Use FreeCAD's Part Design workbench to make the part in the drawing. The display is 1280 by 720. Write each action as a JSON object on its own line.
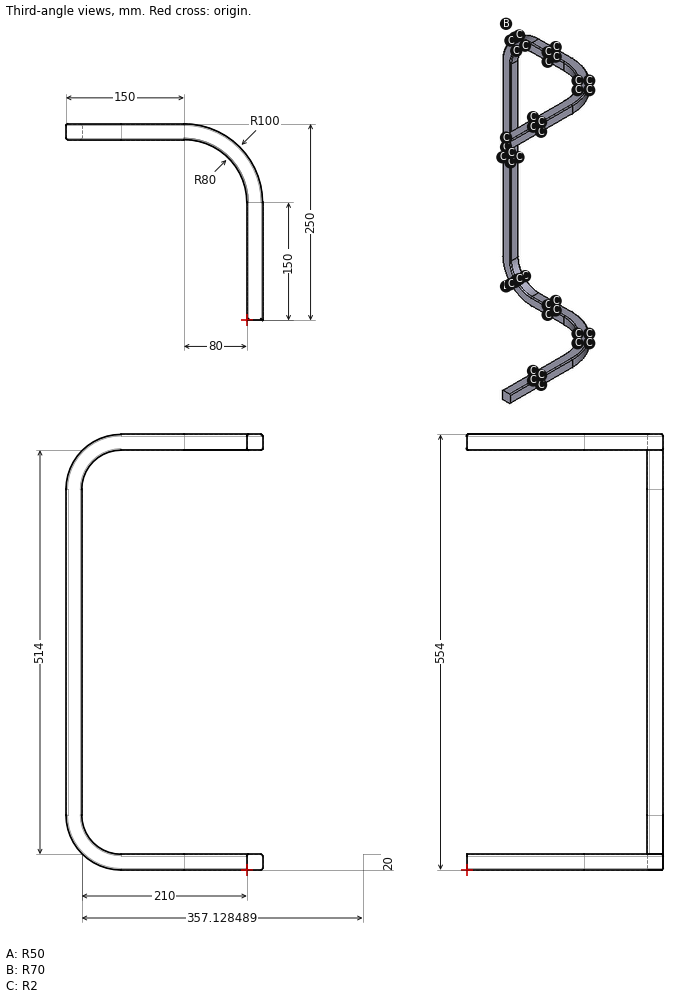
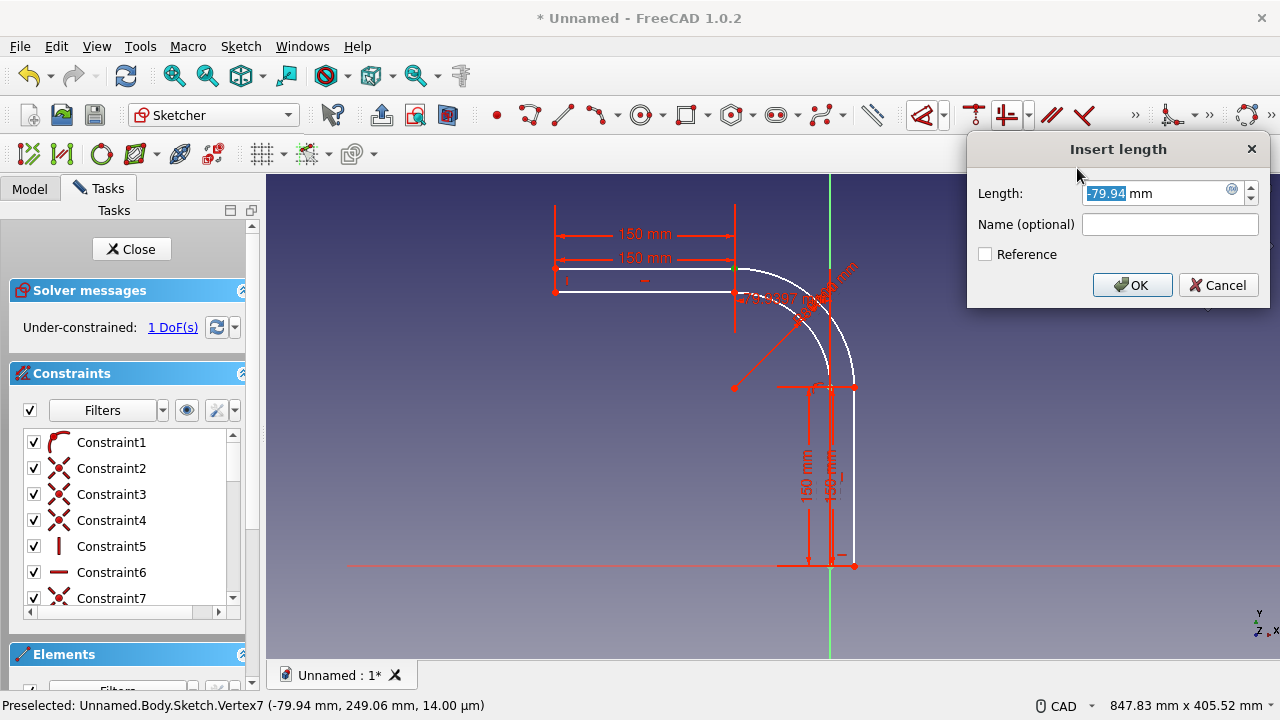
{"action": "type", "text": "-80"}
{"action": "key", "text": "Return"}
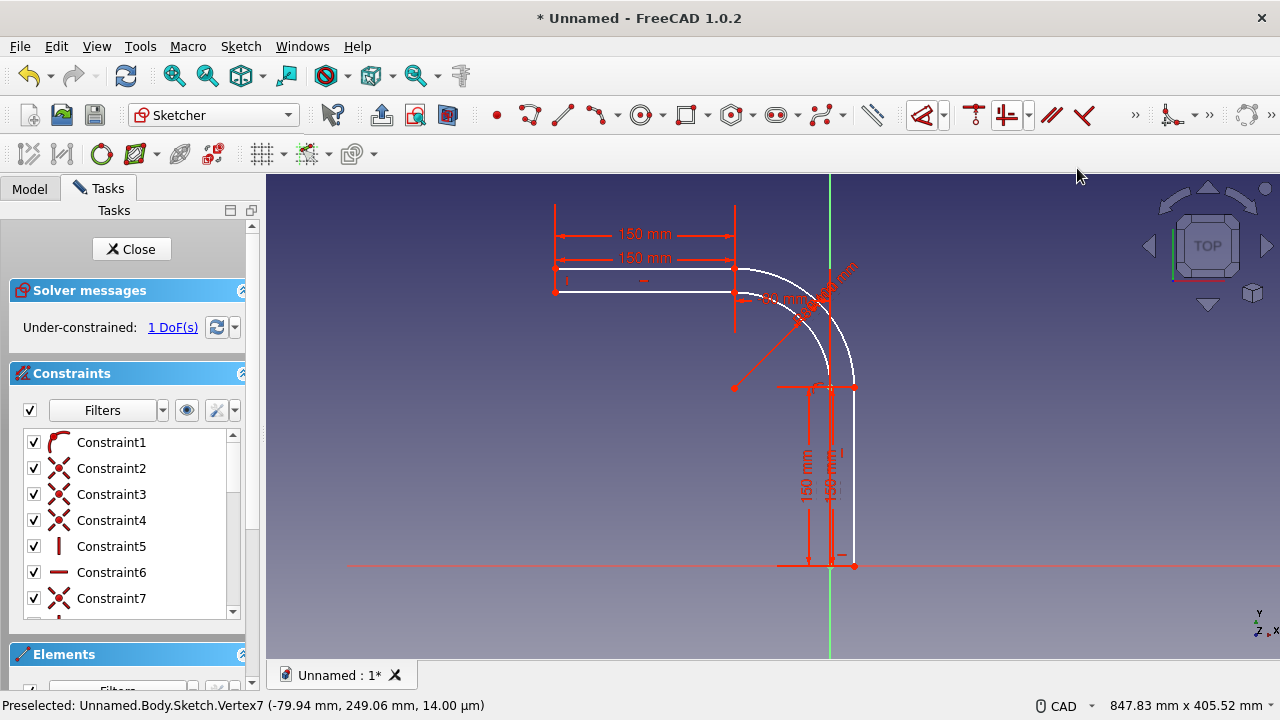
{"action": "left_click", "coordinate": [735, 269]}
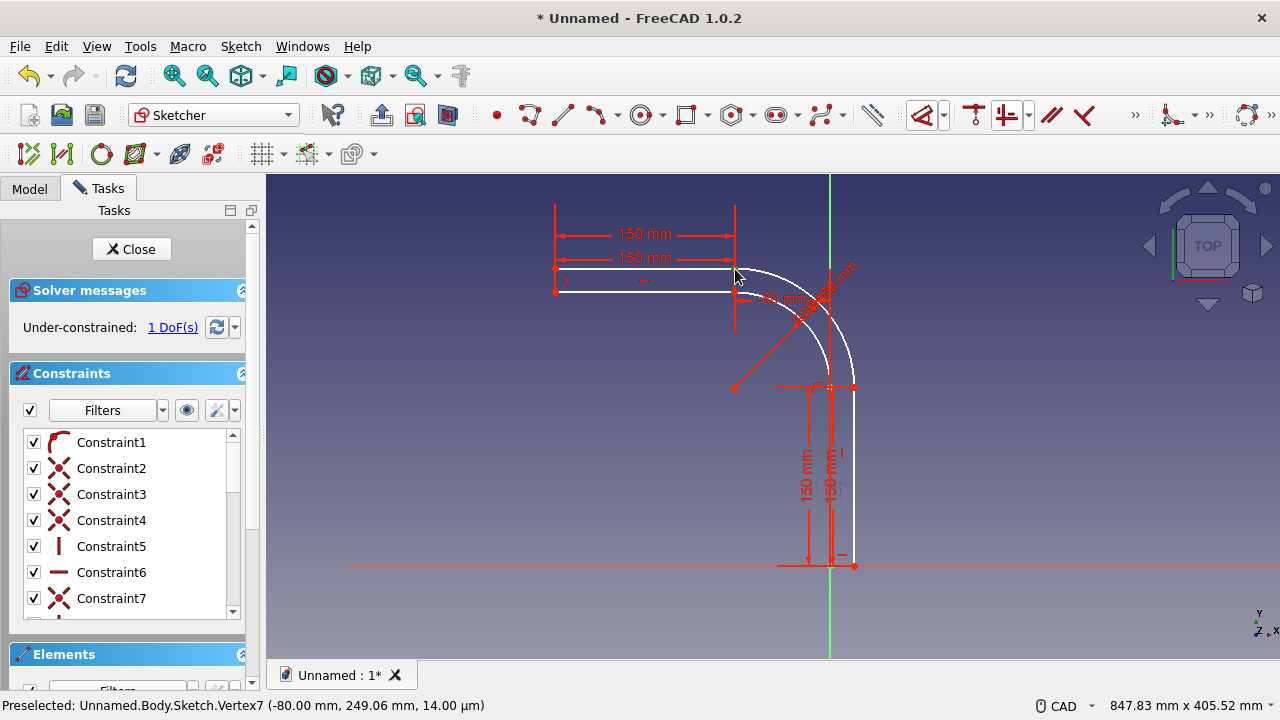
{"action": "key", "text": "i"}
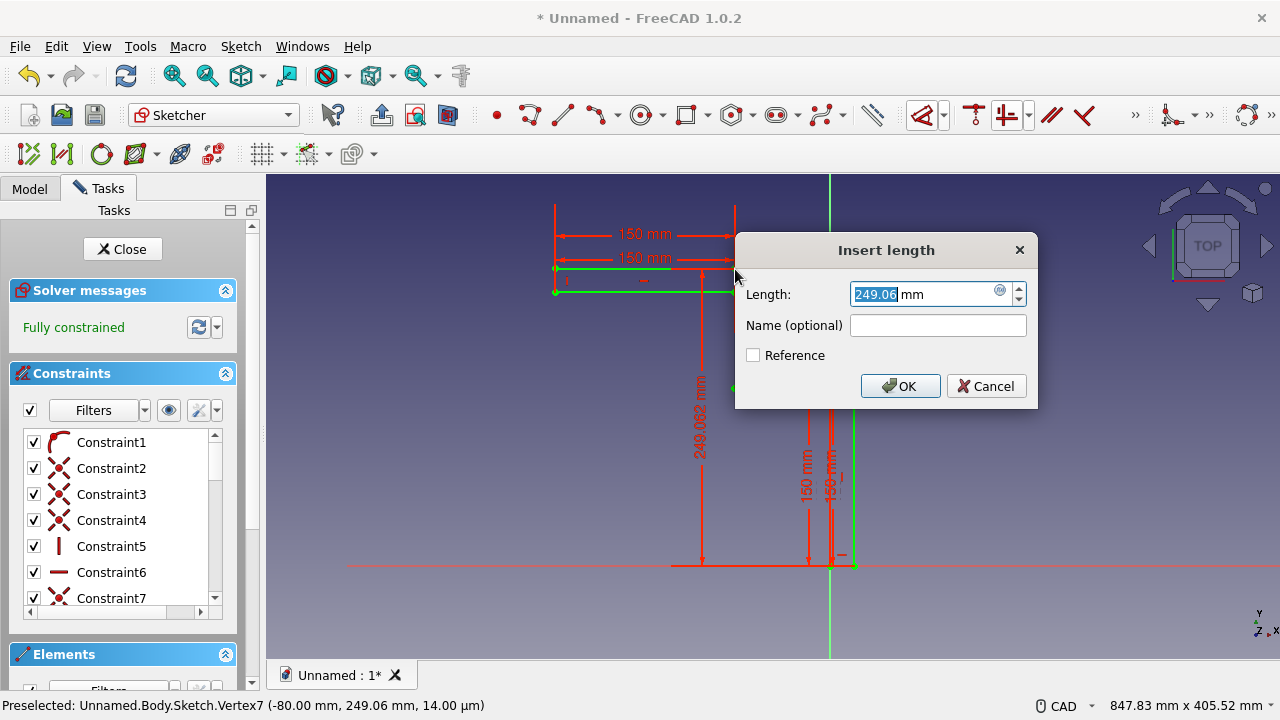
{"action": "type", "text": "250"}
{"action": "key", "text": "Return"}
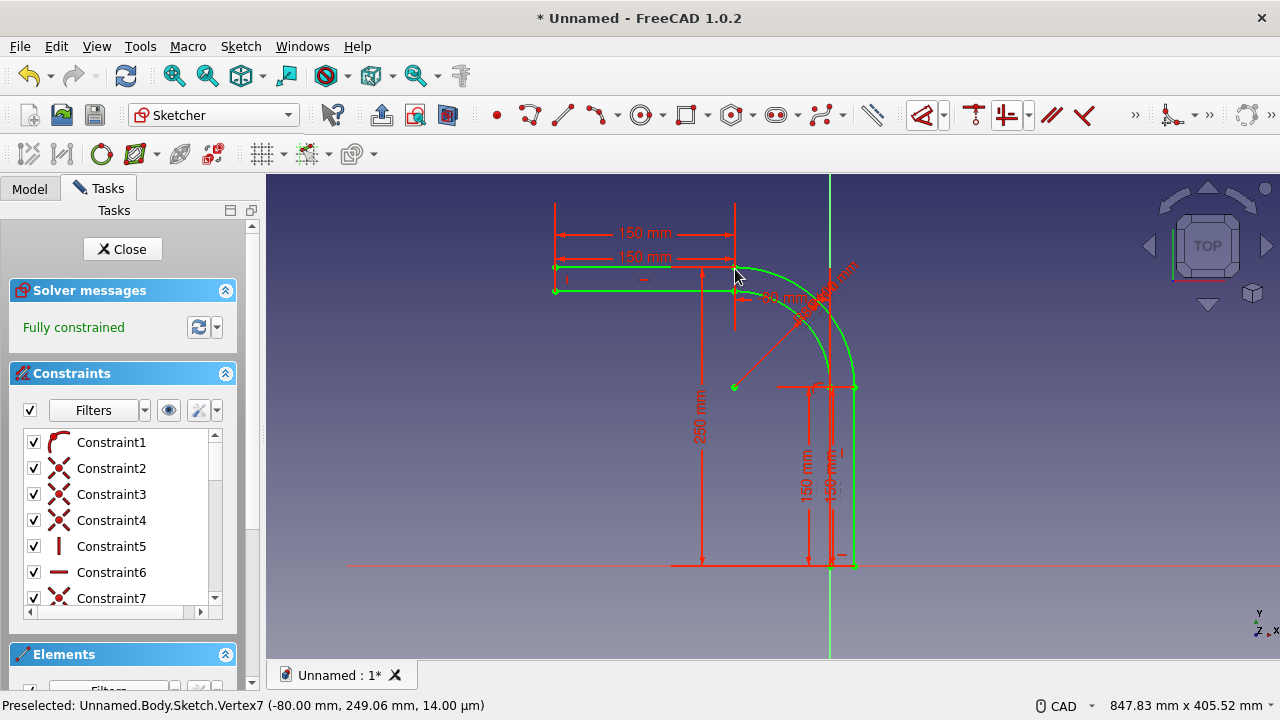
{"action": "left_click", "coordinate": [123, 249]}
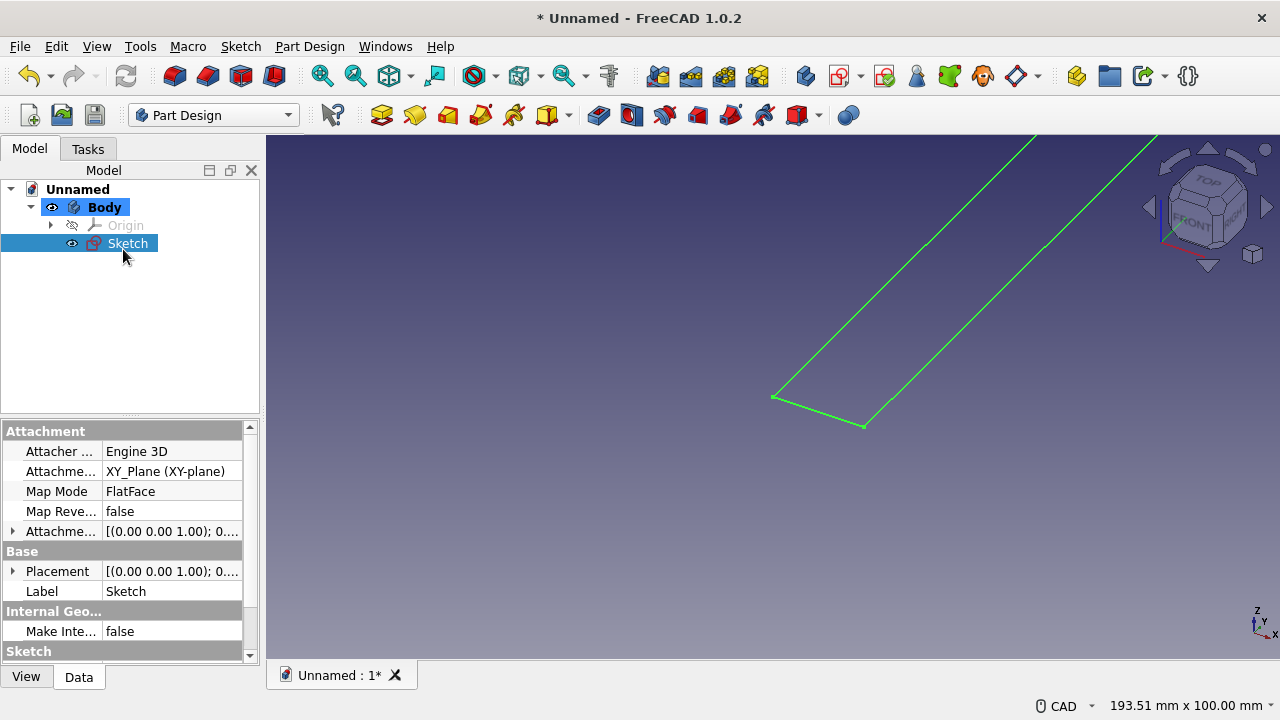
{"action": "left_click", "coordinate": [382, 116]}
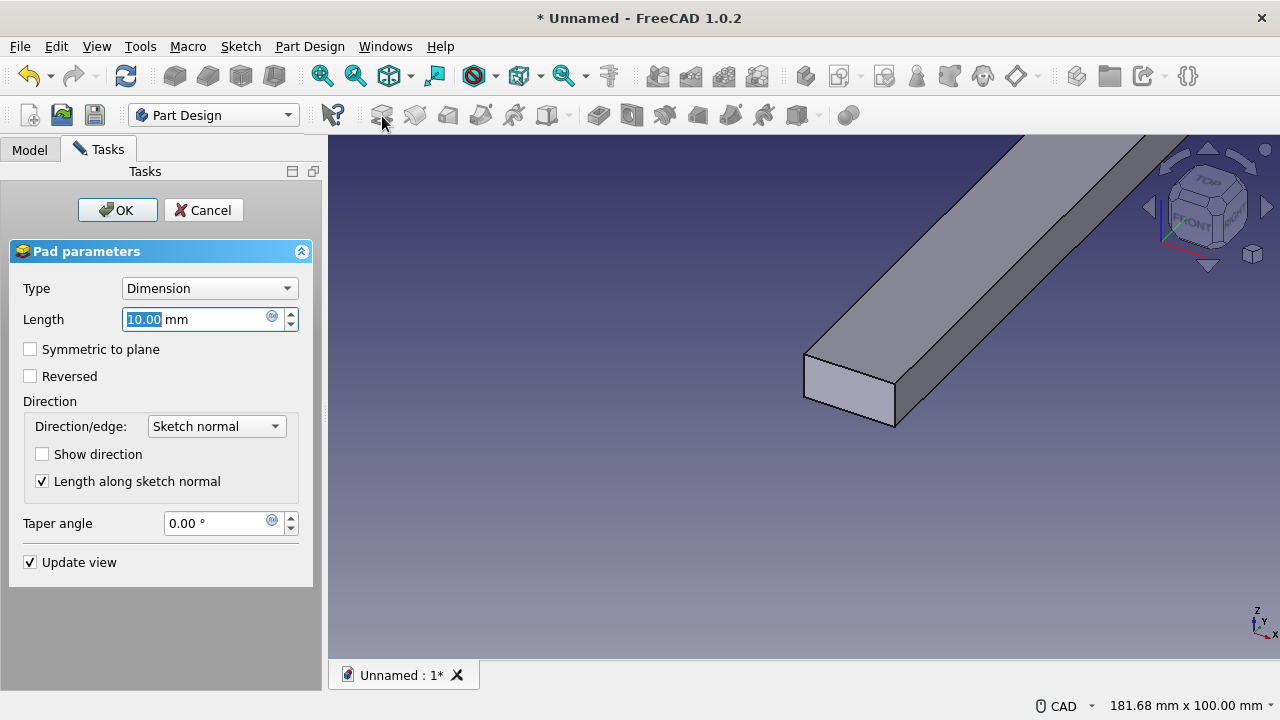
{"action": "type", "text": "554"}
{"action": "key", "text": "Tab"}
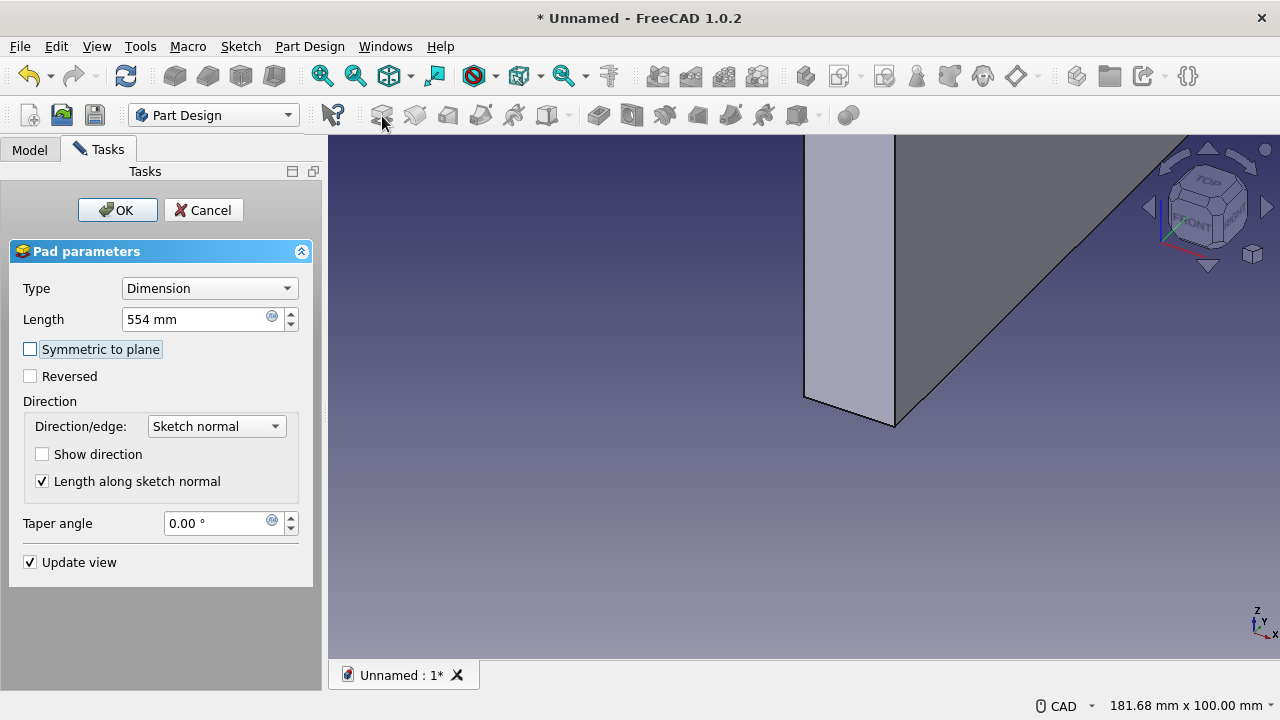
{"action": "left_click", "coordinate": [118, 210]}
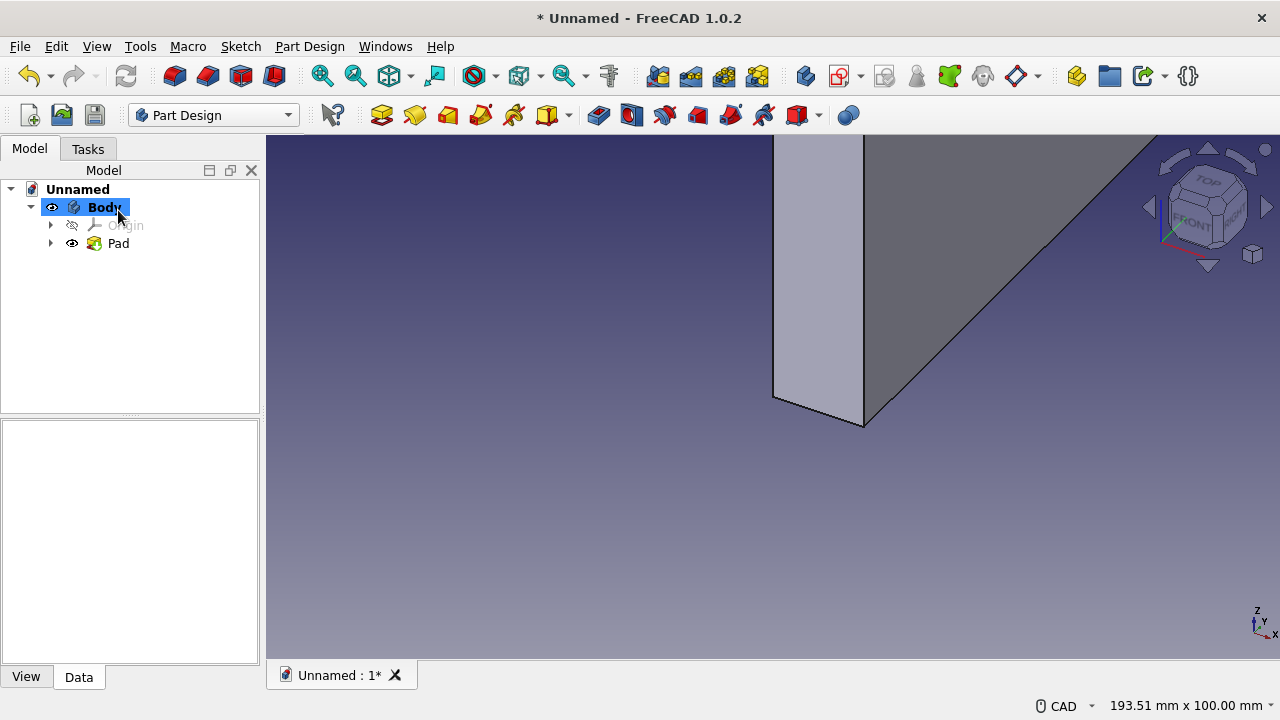
{"action": "left_click", "coordinate": [323, 76]}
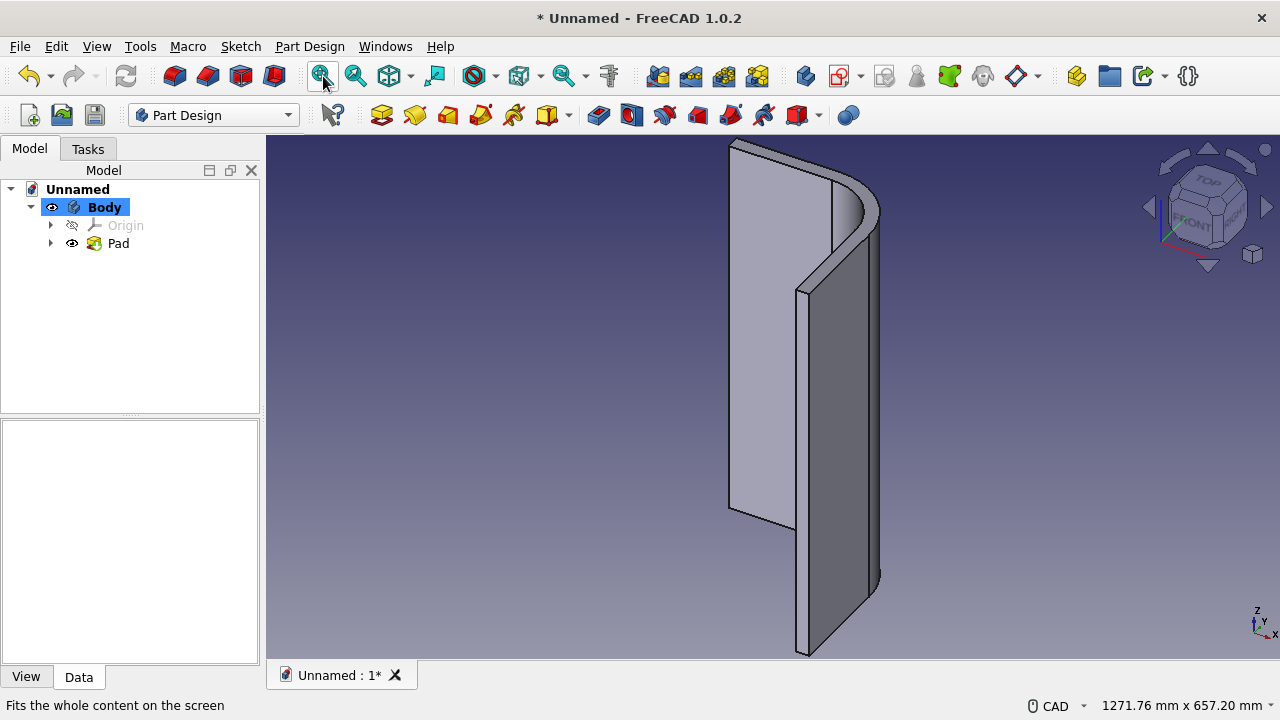
{"action": "key", "text": "4"}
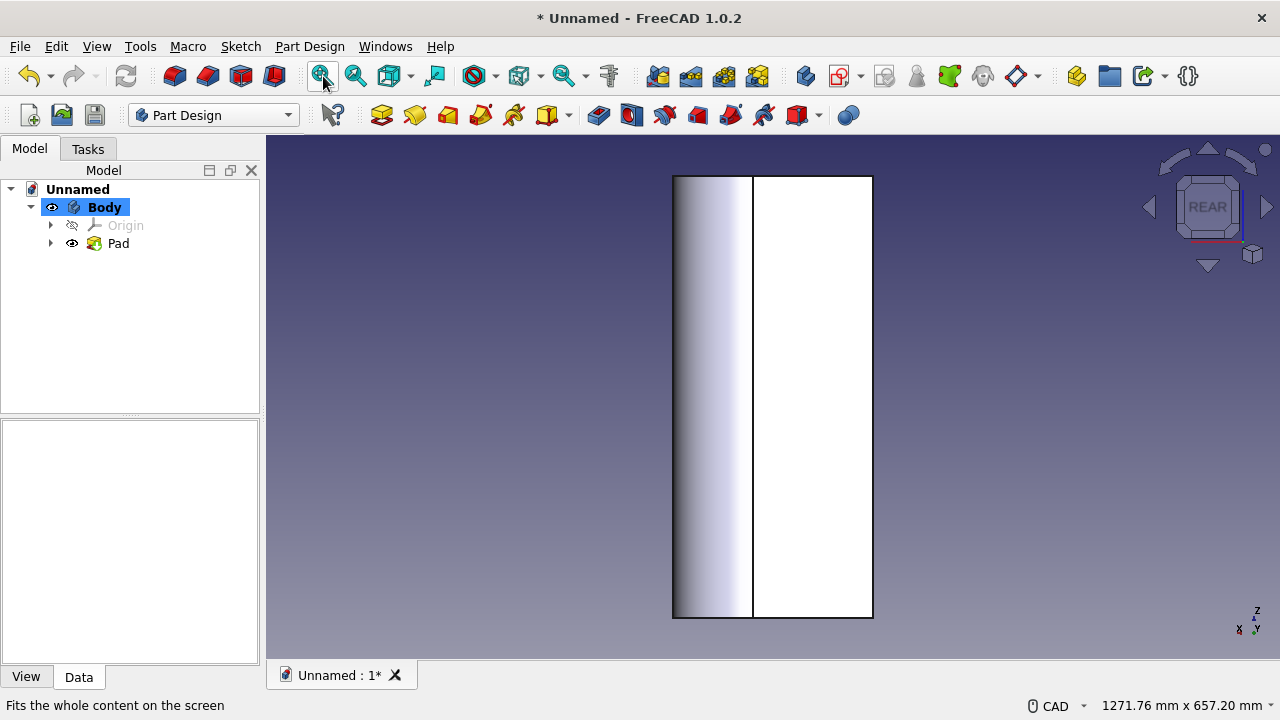
{"action": "left_click", "coordinate": [813, 270]}